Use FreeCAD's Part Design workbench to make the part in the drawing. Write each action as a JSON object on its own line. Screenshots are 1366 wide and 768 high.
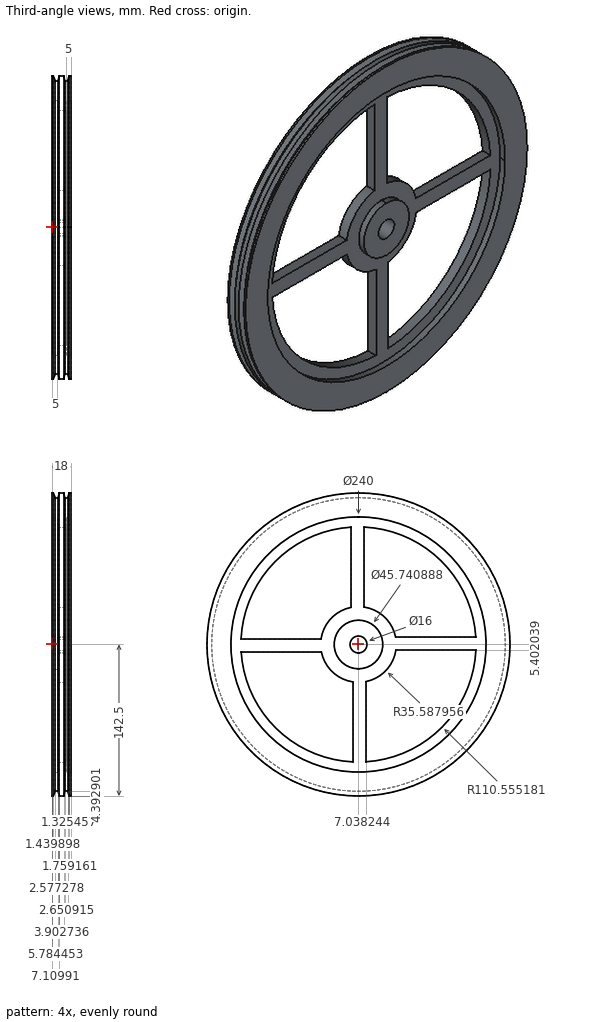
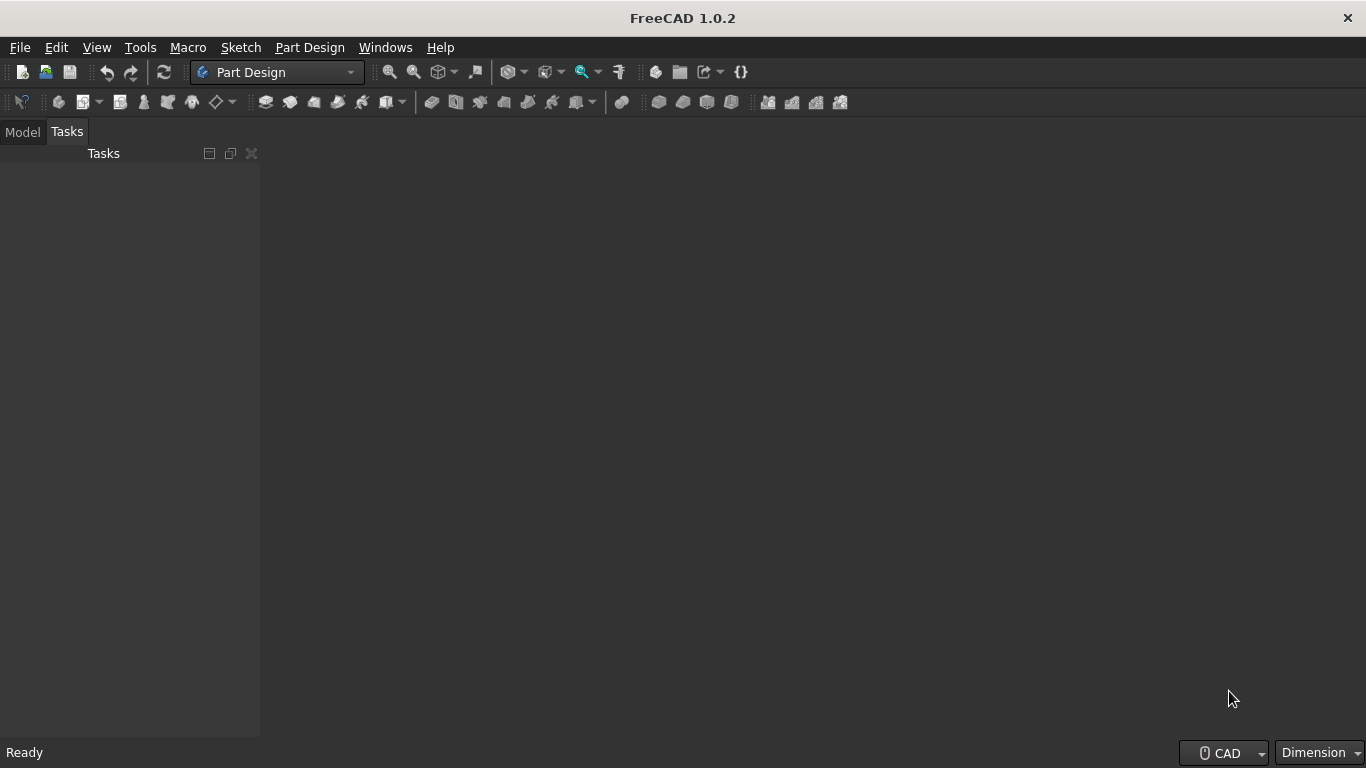
{"action": "key", "text": "ctrl+n"}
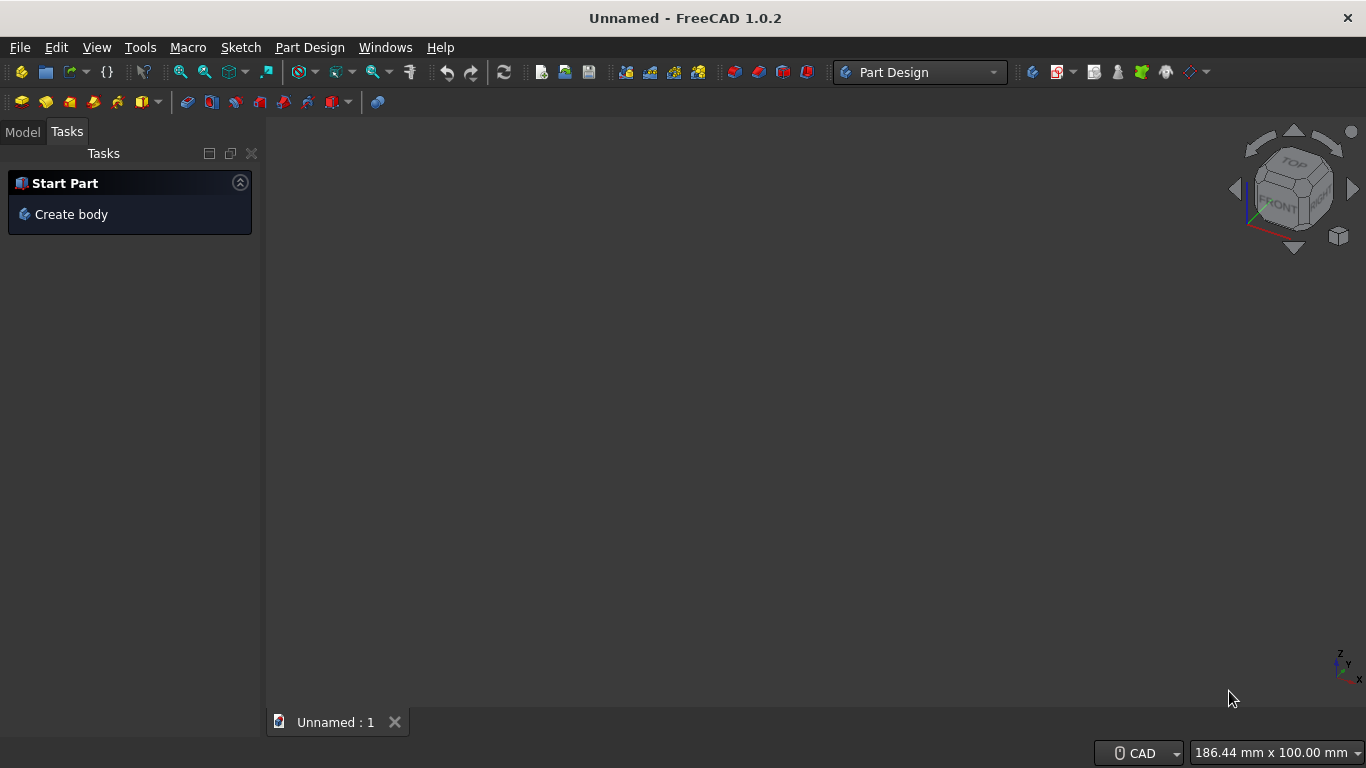
{"action": "left_click", "coordinate": [1058, 72]}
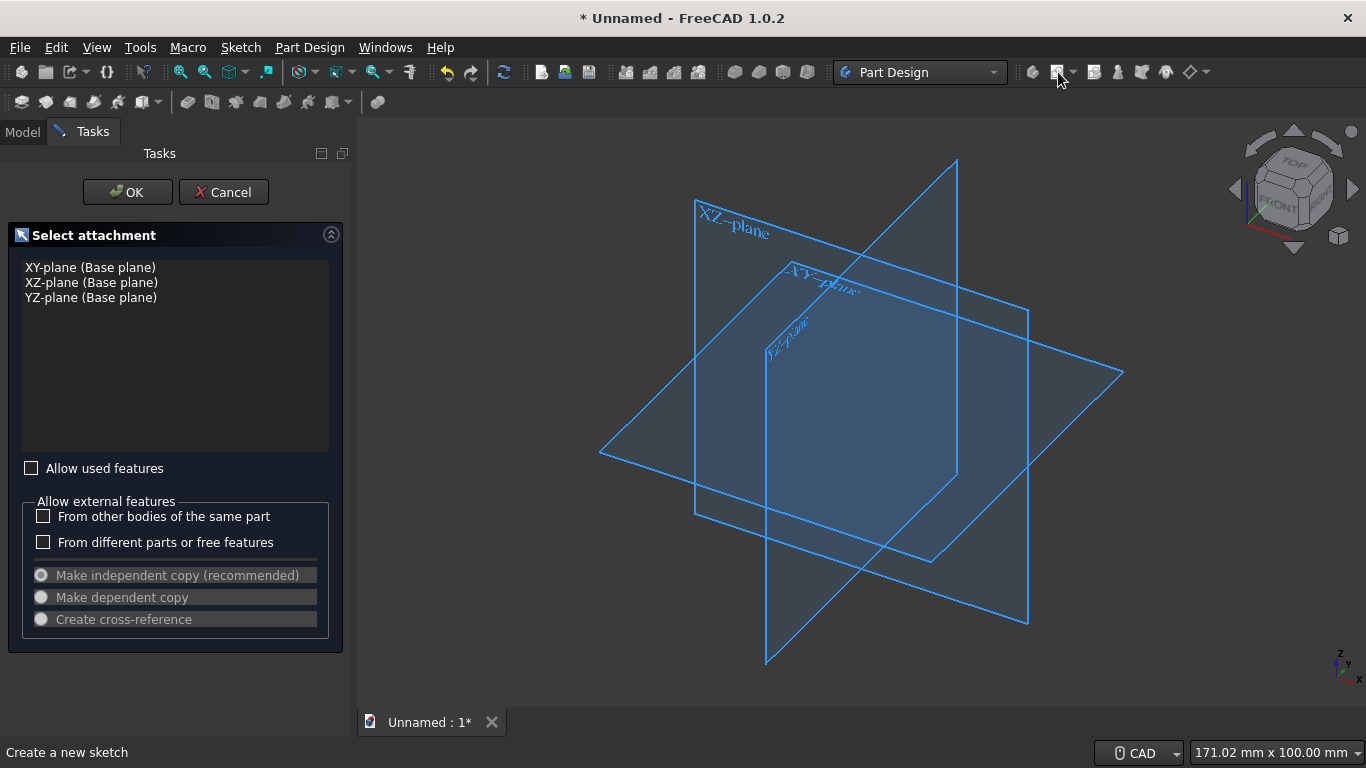
{"action": "left_click", "coordinate": [82, 282]}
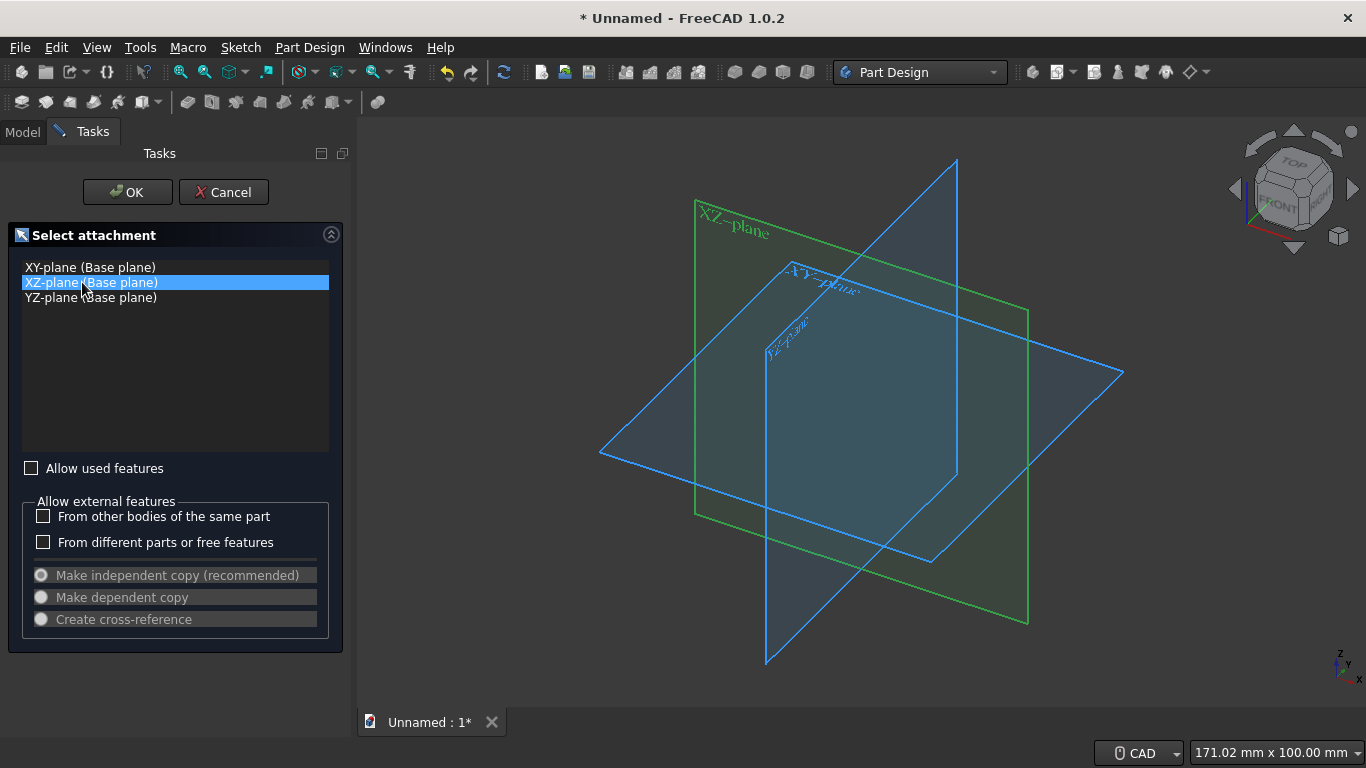
{"action": "left_click", "coordinate": [128, 192]}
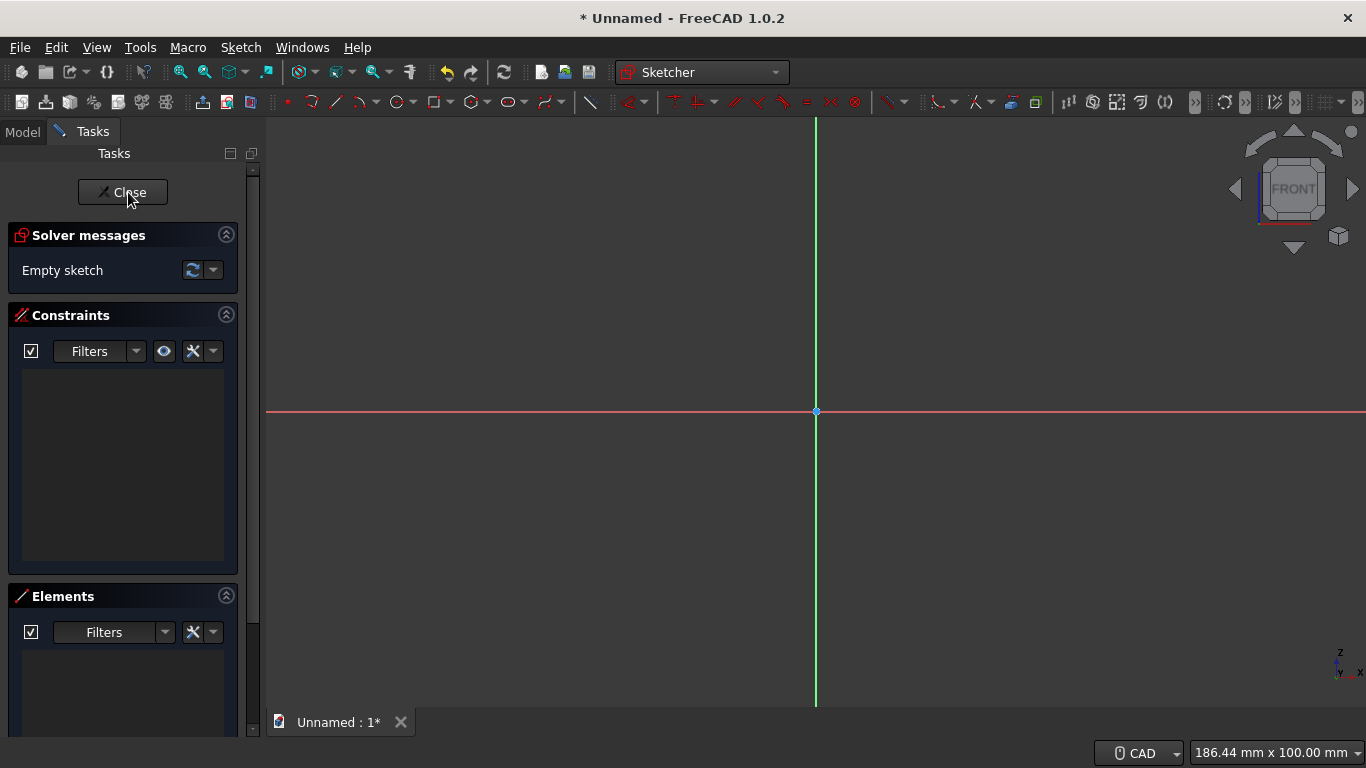
{"action": "scroll", "coordinate": [648, 145], "scroll_direction": "down", "scroll_amount": 4}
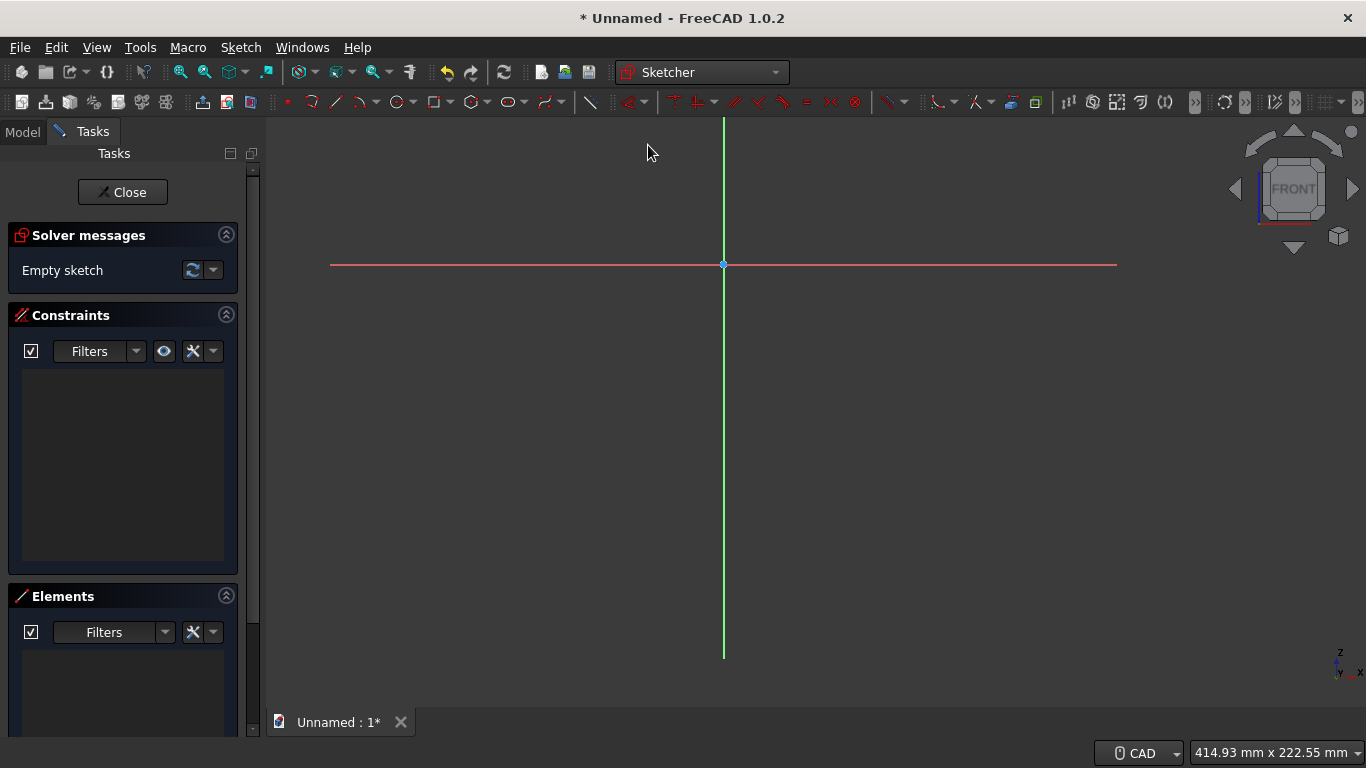
{"action": "key", "text": "g m"}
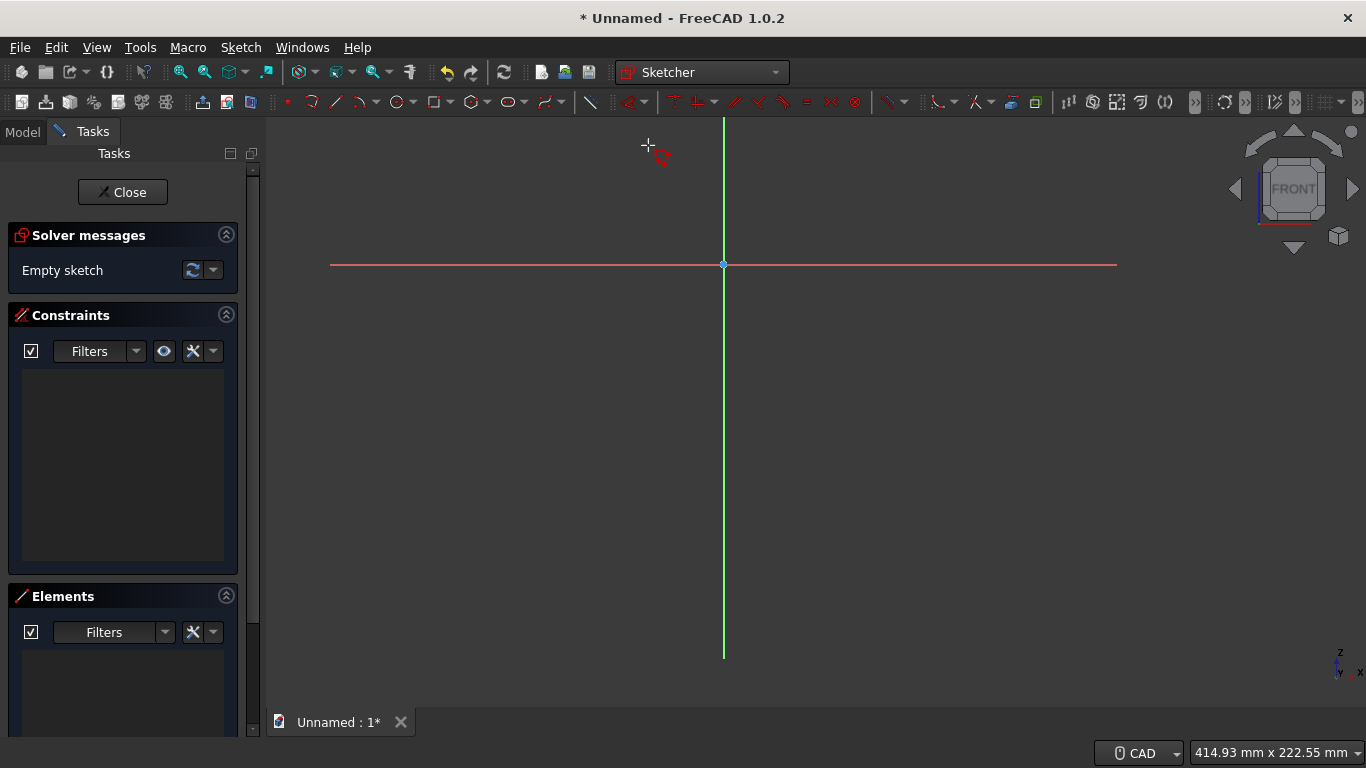
{"action": "left_click", "coordinate": [724, 265]}
{"action": "left_click", "coordinate": [771, 274]}
{"action": "left_click", "coordinate": [771, 643]}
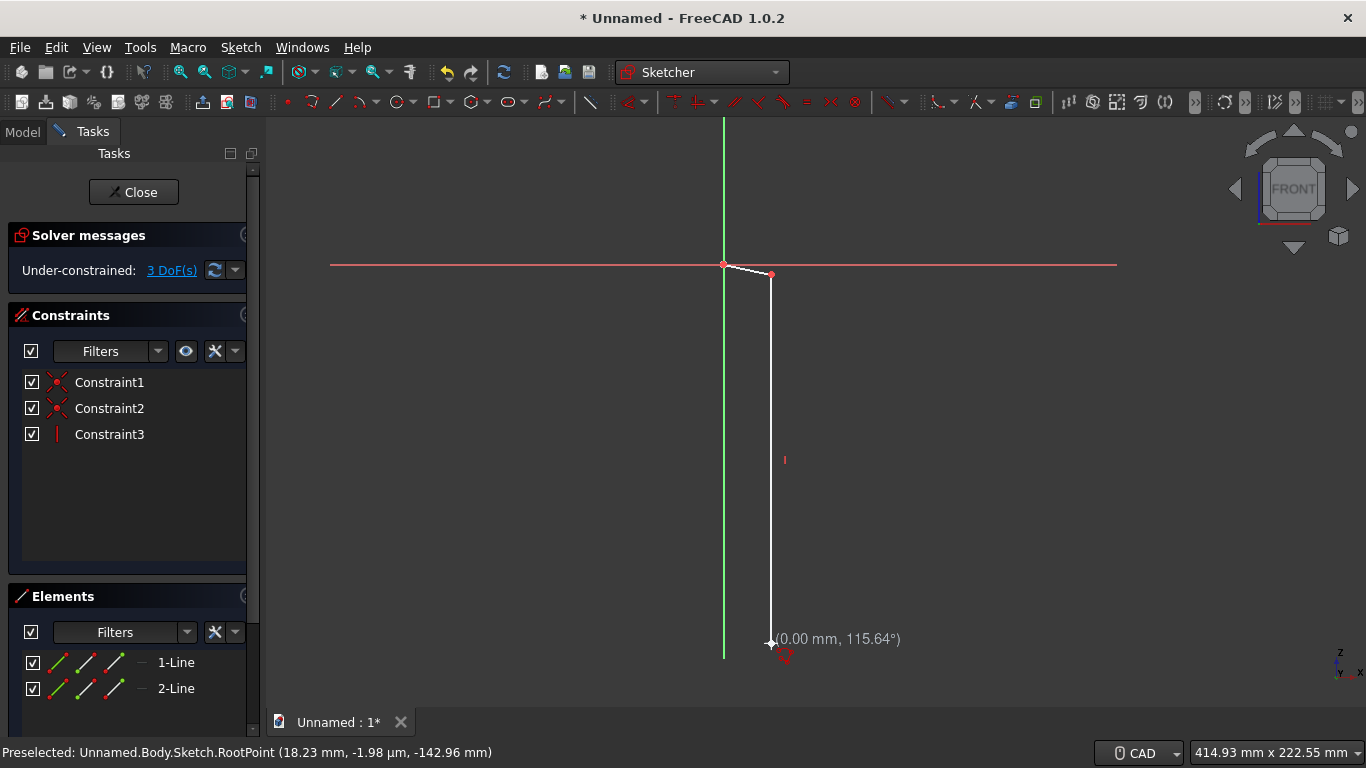
{"action": "scroll", "coordinate": [767, 643], "scroll_direction": "up", "scroll_amount": 7}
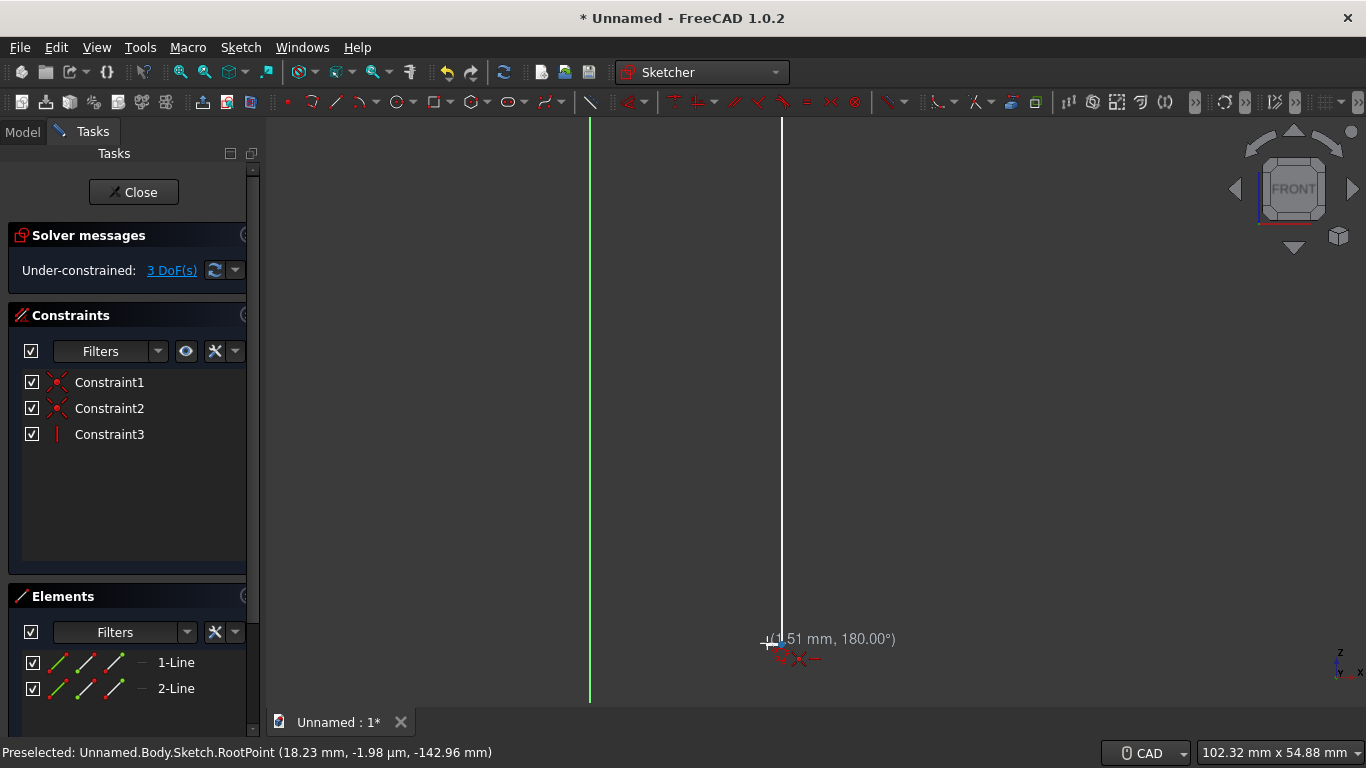
{"action": "left_click", "coordinate": [765, 640]}
{"action": "left_click", "coordinate": [750, 592]}
{"action": "left_click", "coordinate": [722, 592]}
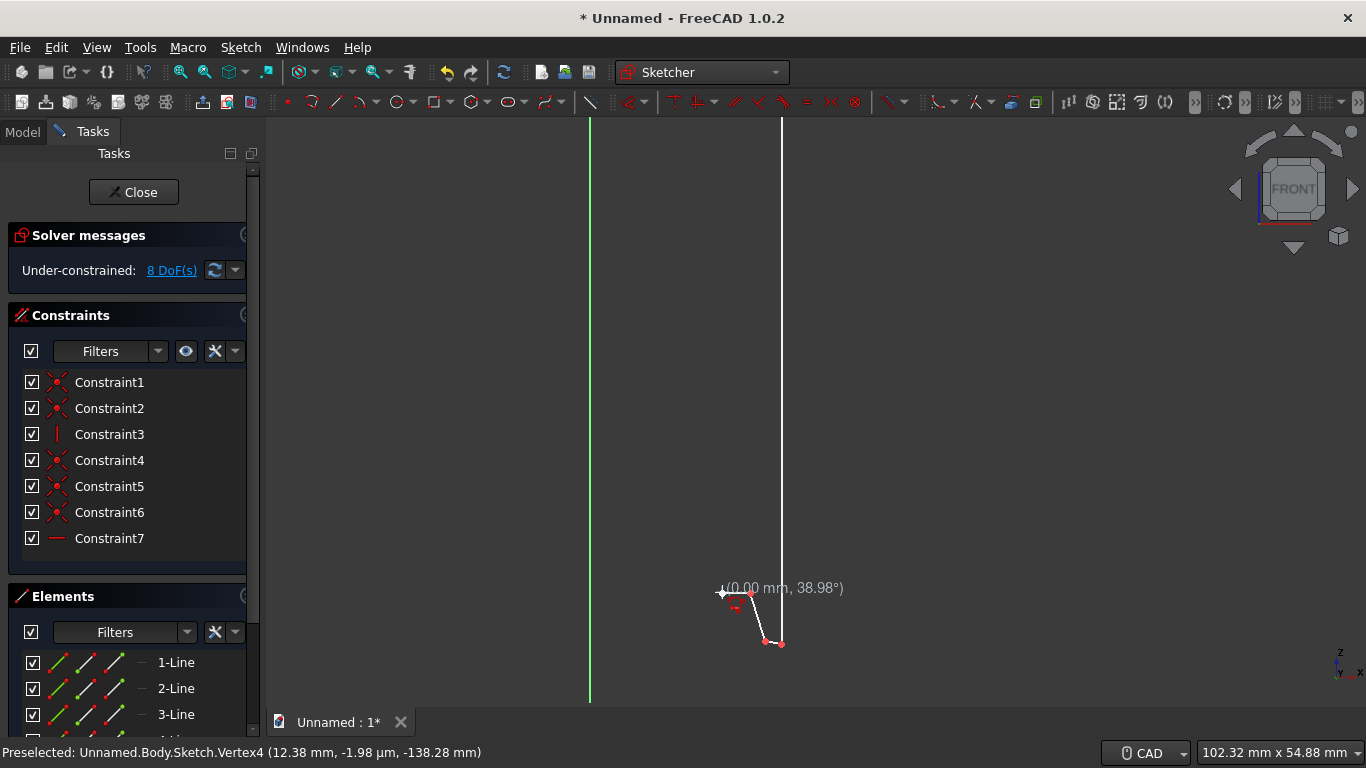
{"action": "scroll", "coordinate": [767, 588], "scroll_direction": "down", "scroll_amount": 7}